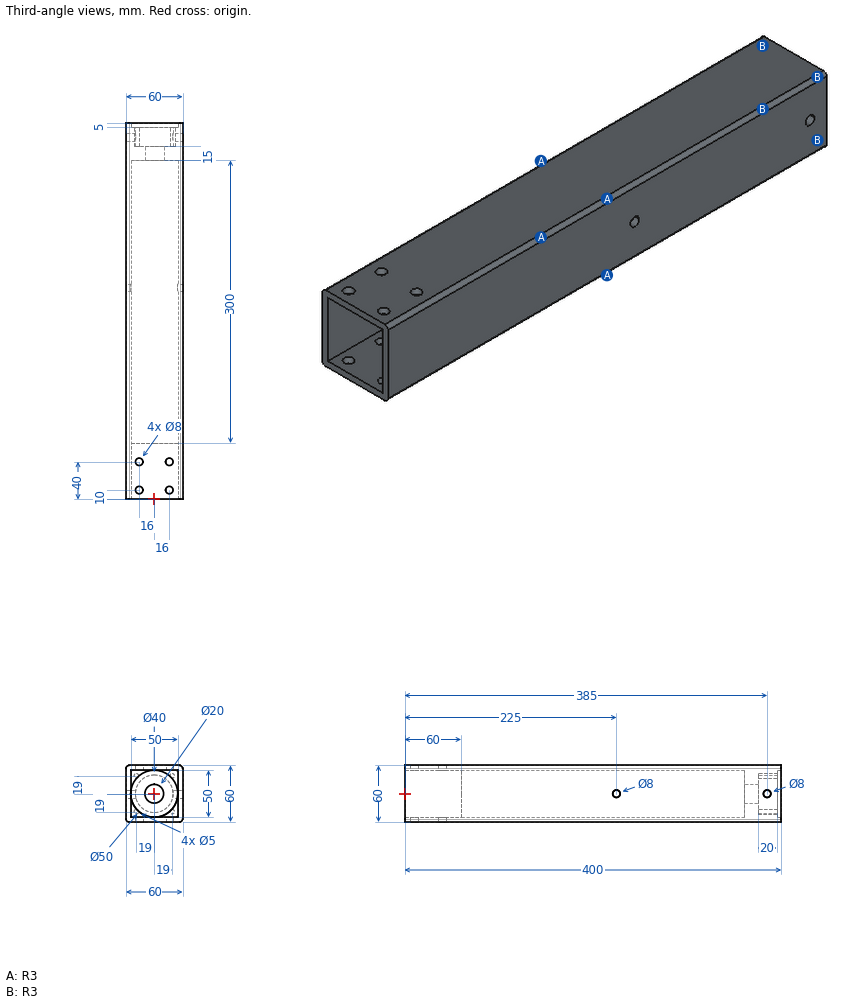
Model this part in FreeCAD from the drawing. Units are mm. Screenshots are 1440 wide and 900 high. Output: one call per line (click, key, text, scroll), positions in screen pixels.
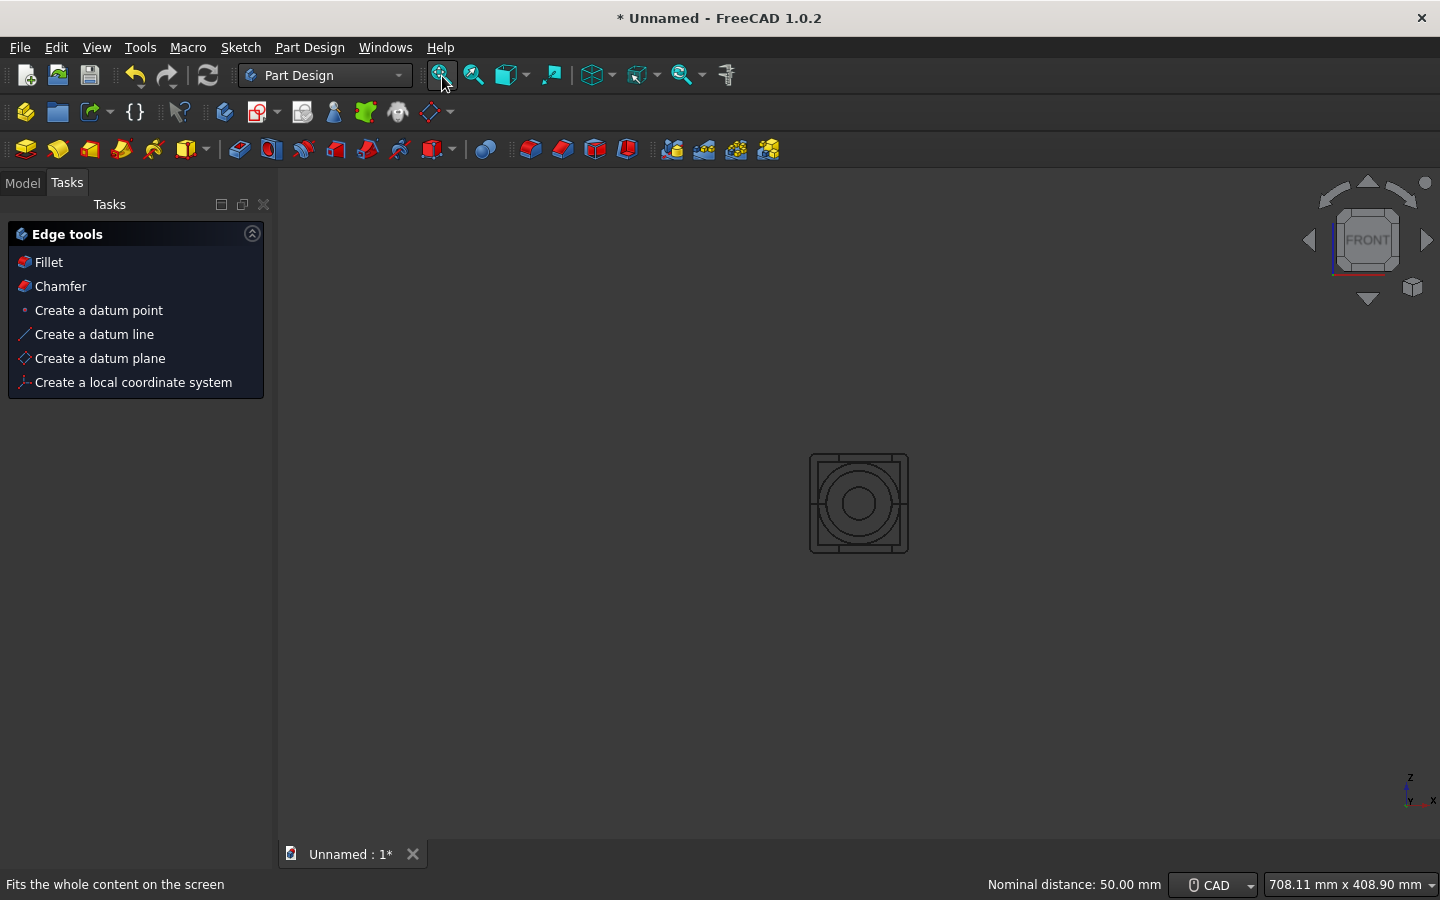
click(442, 76)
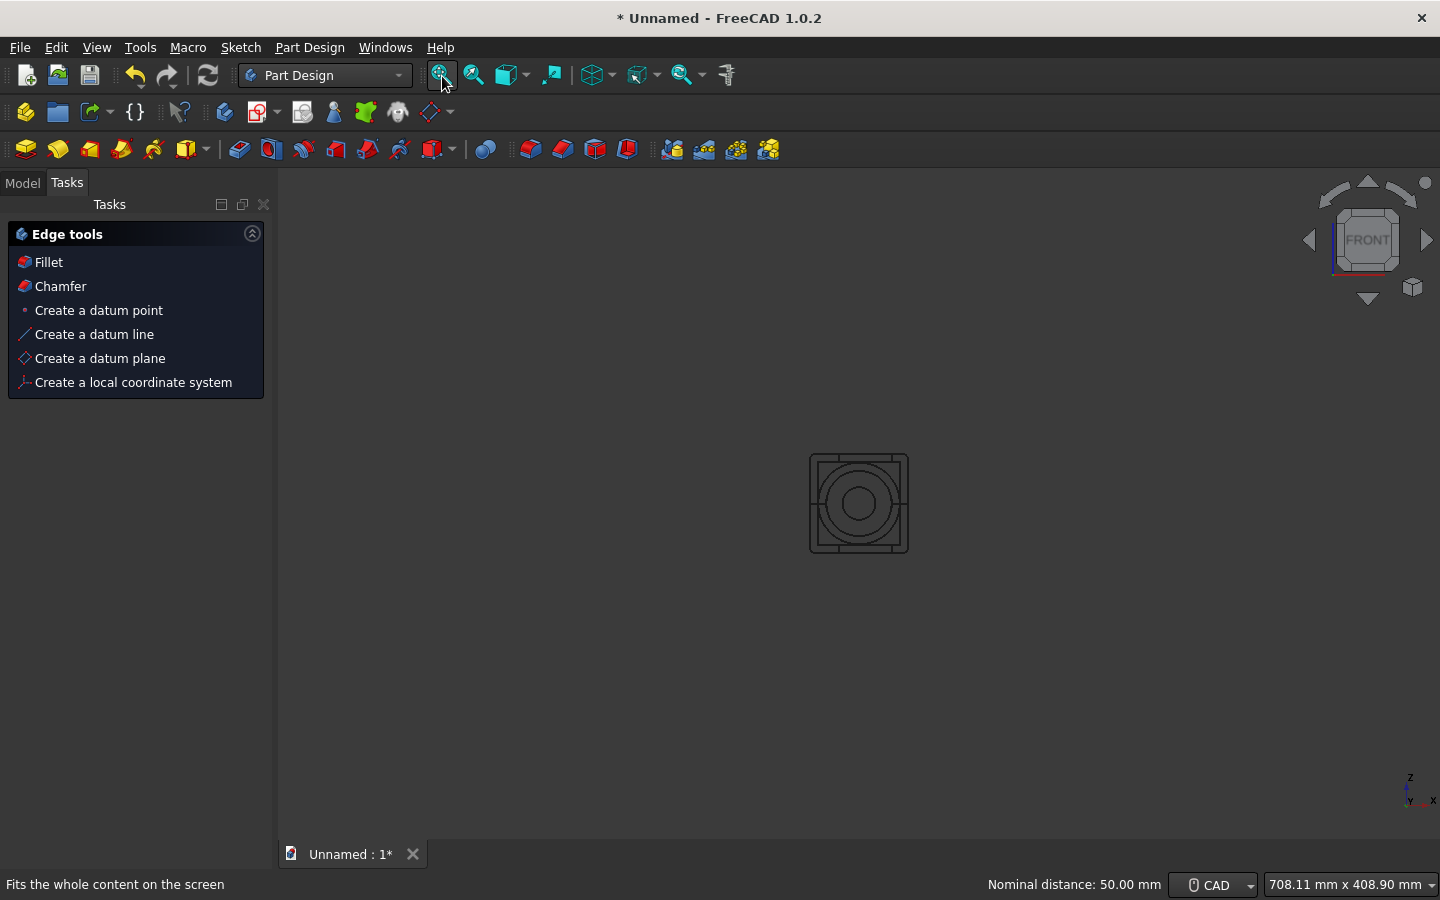
scroll(900, 461, up, 8)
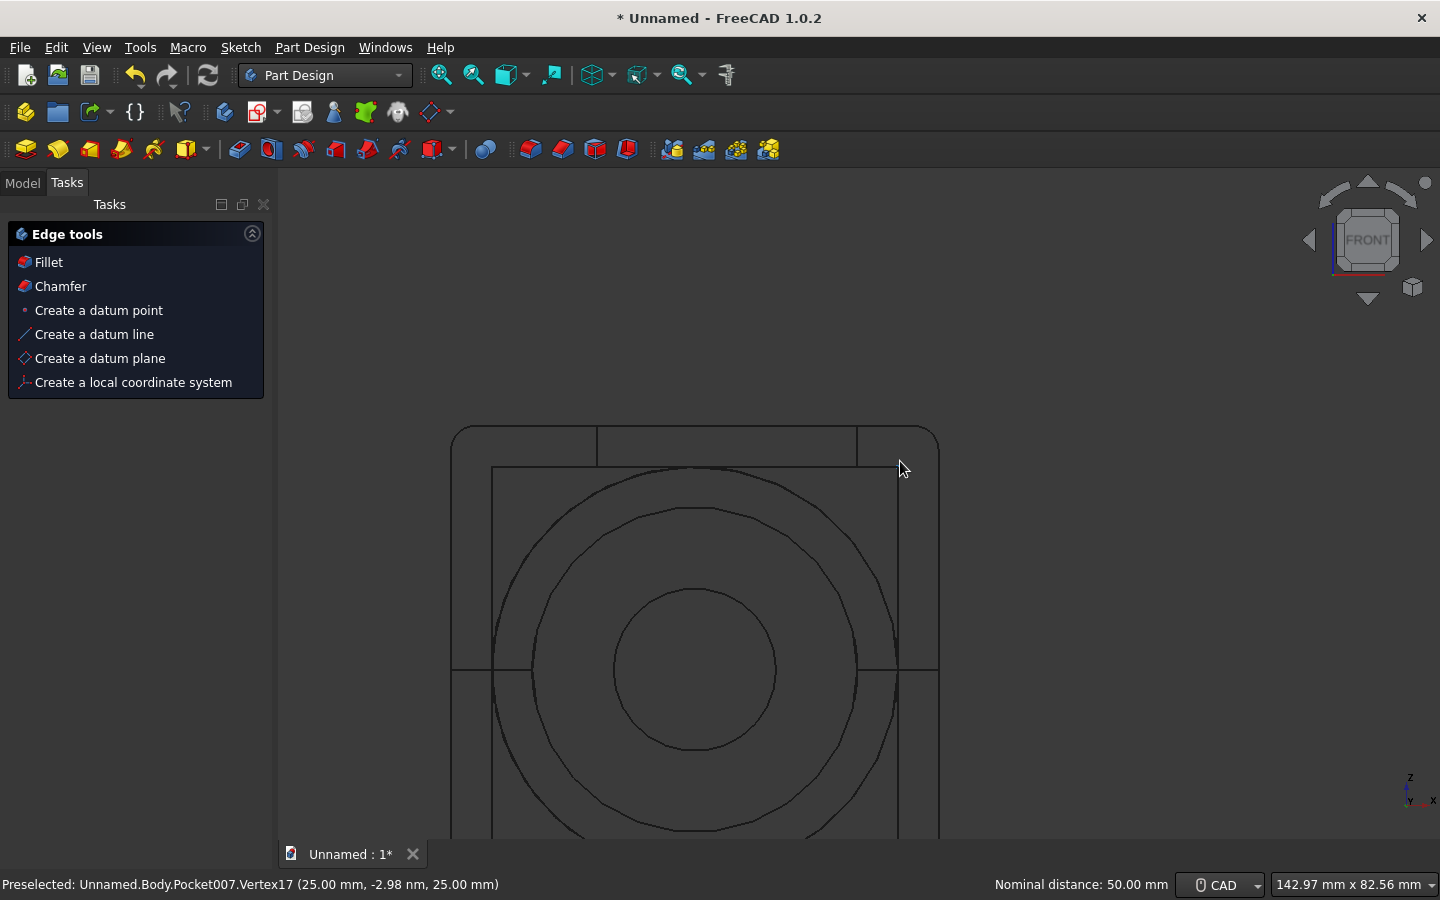
click(442, 76)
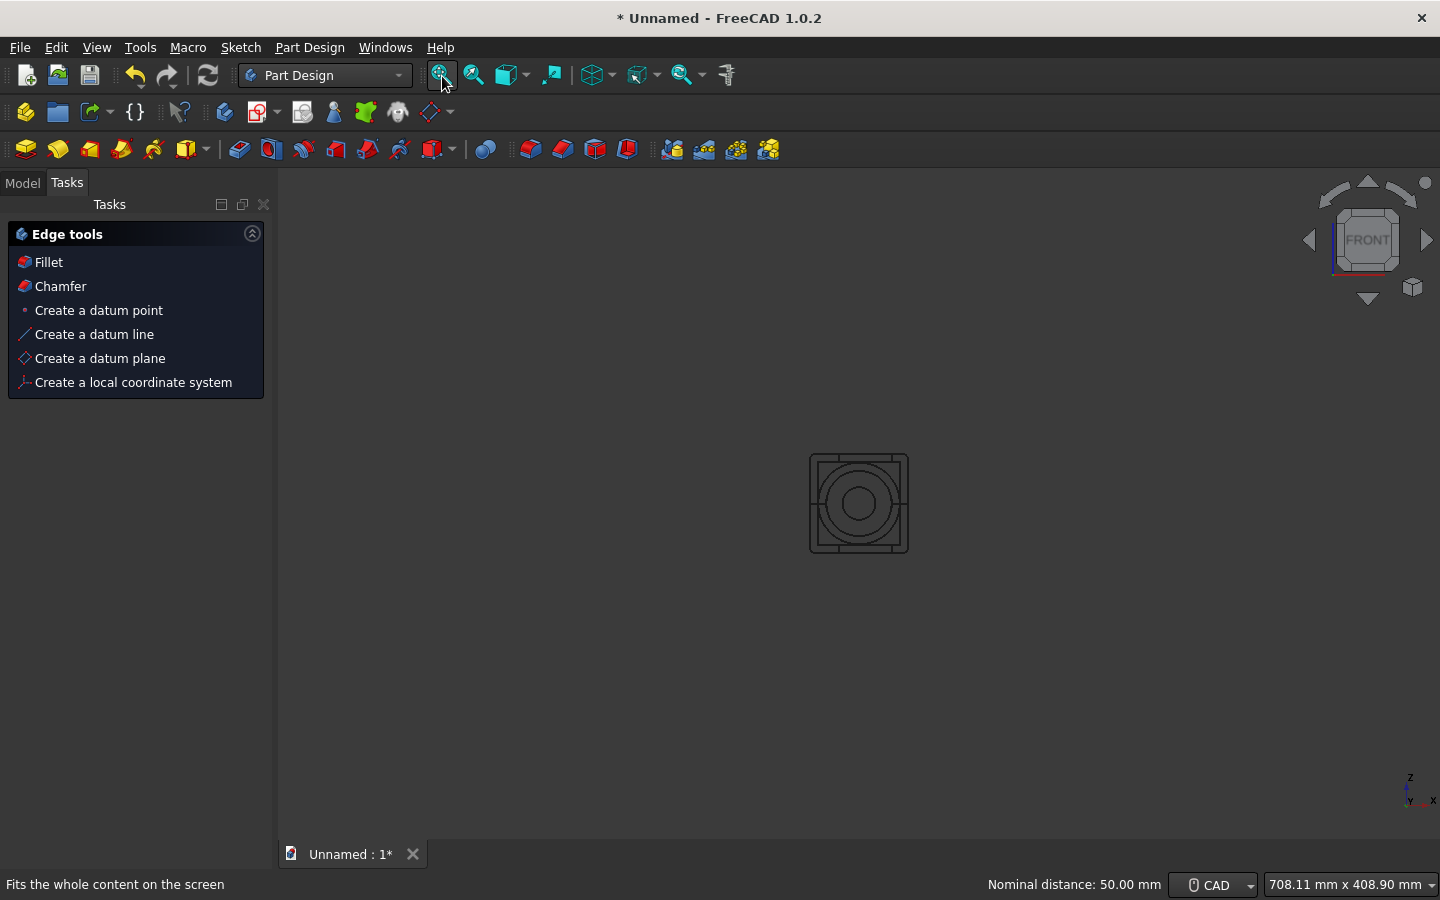
key(3)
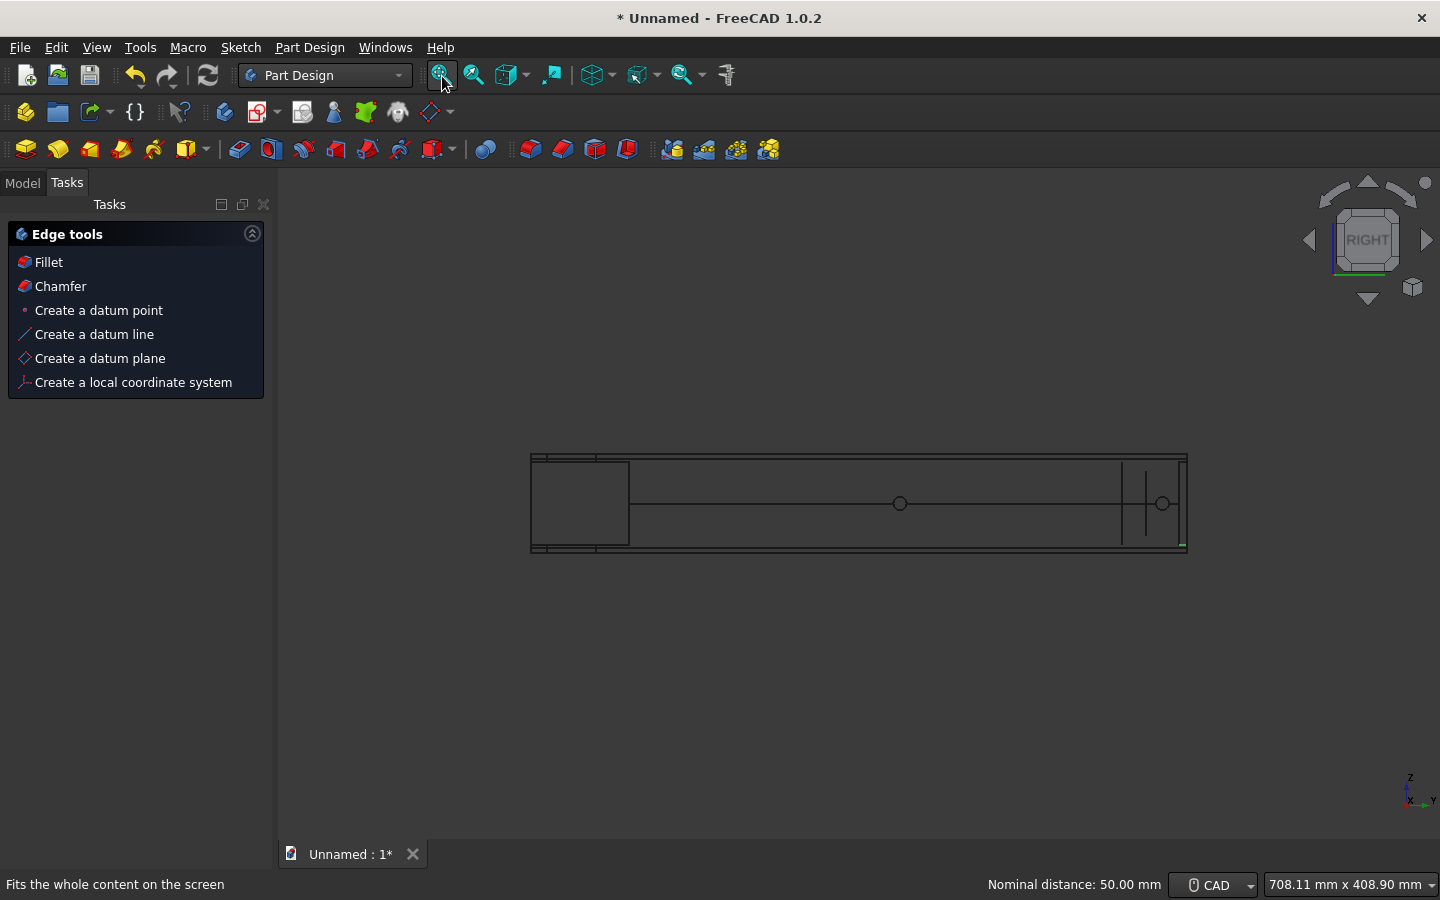
scroll(1183, 461, up, 8)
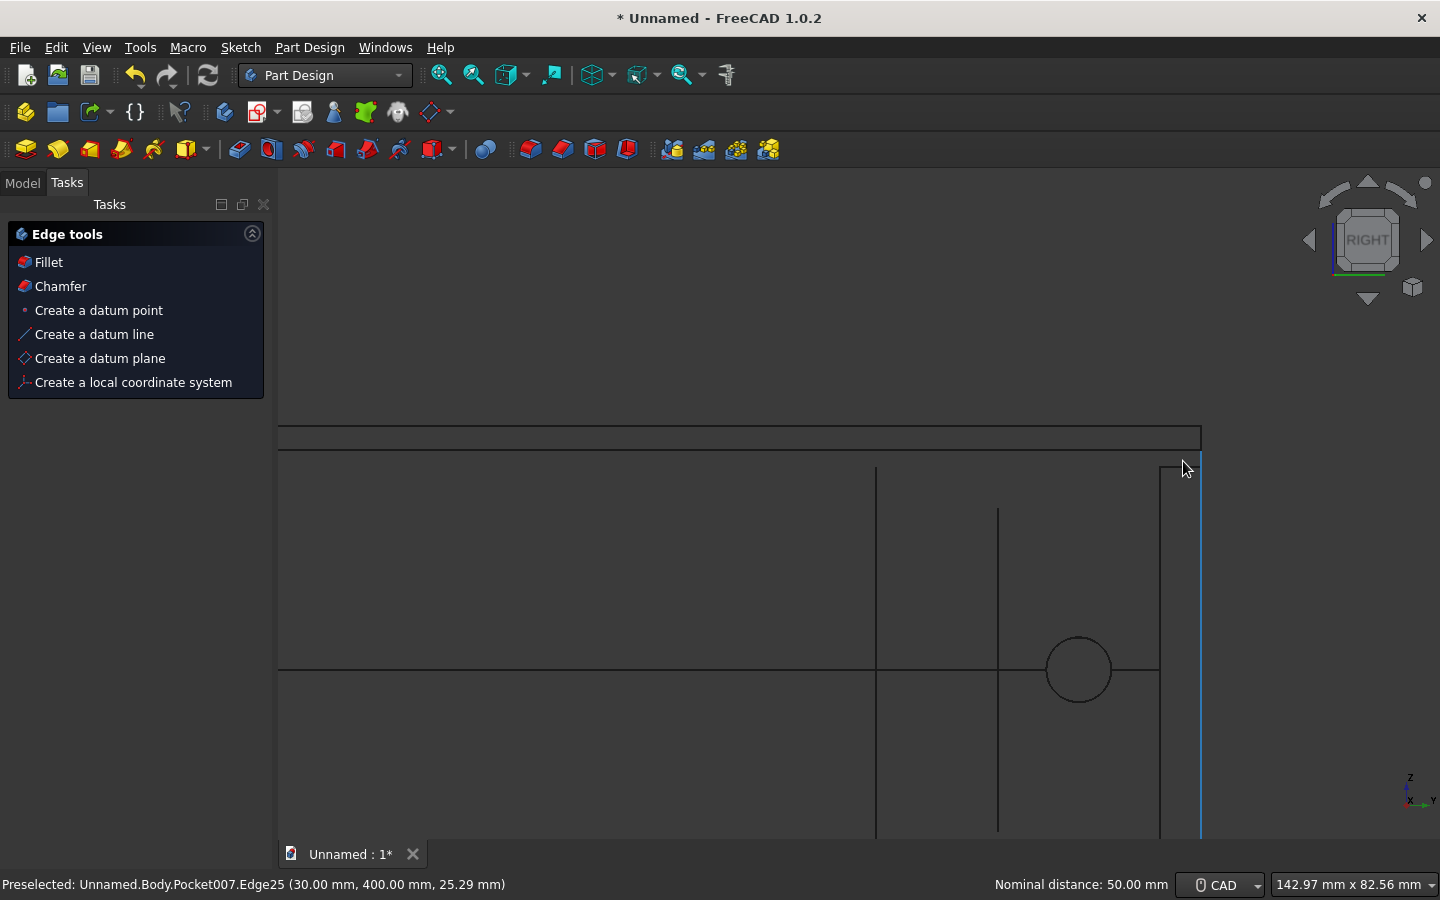
click(1180, 466, ctrl)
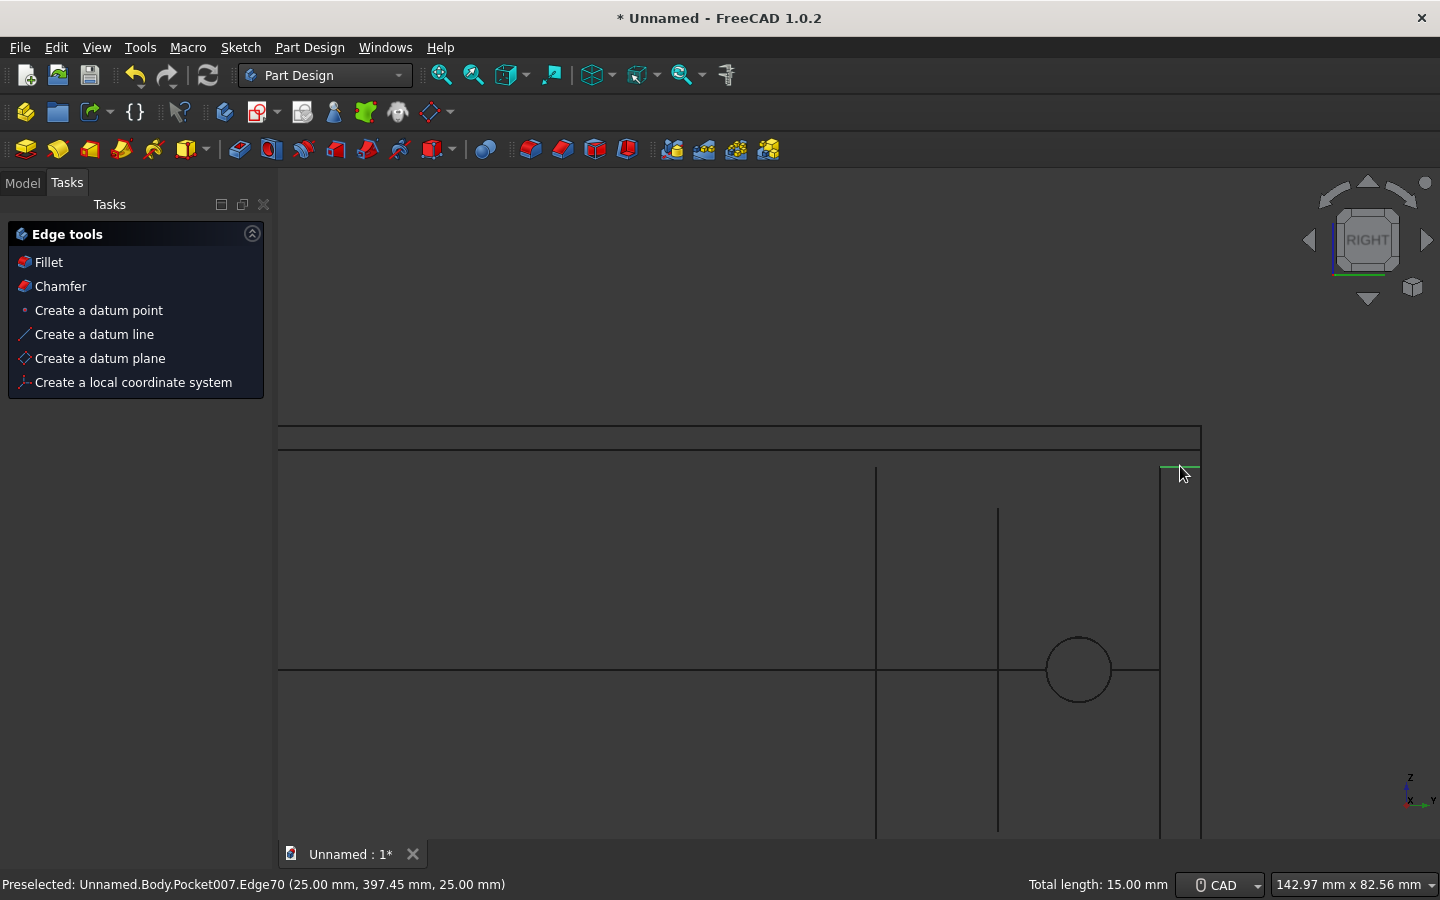
key(v)
key(f)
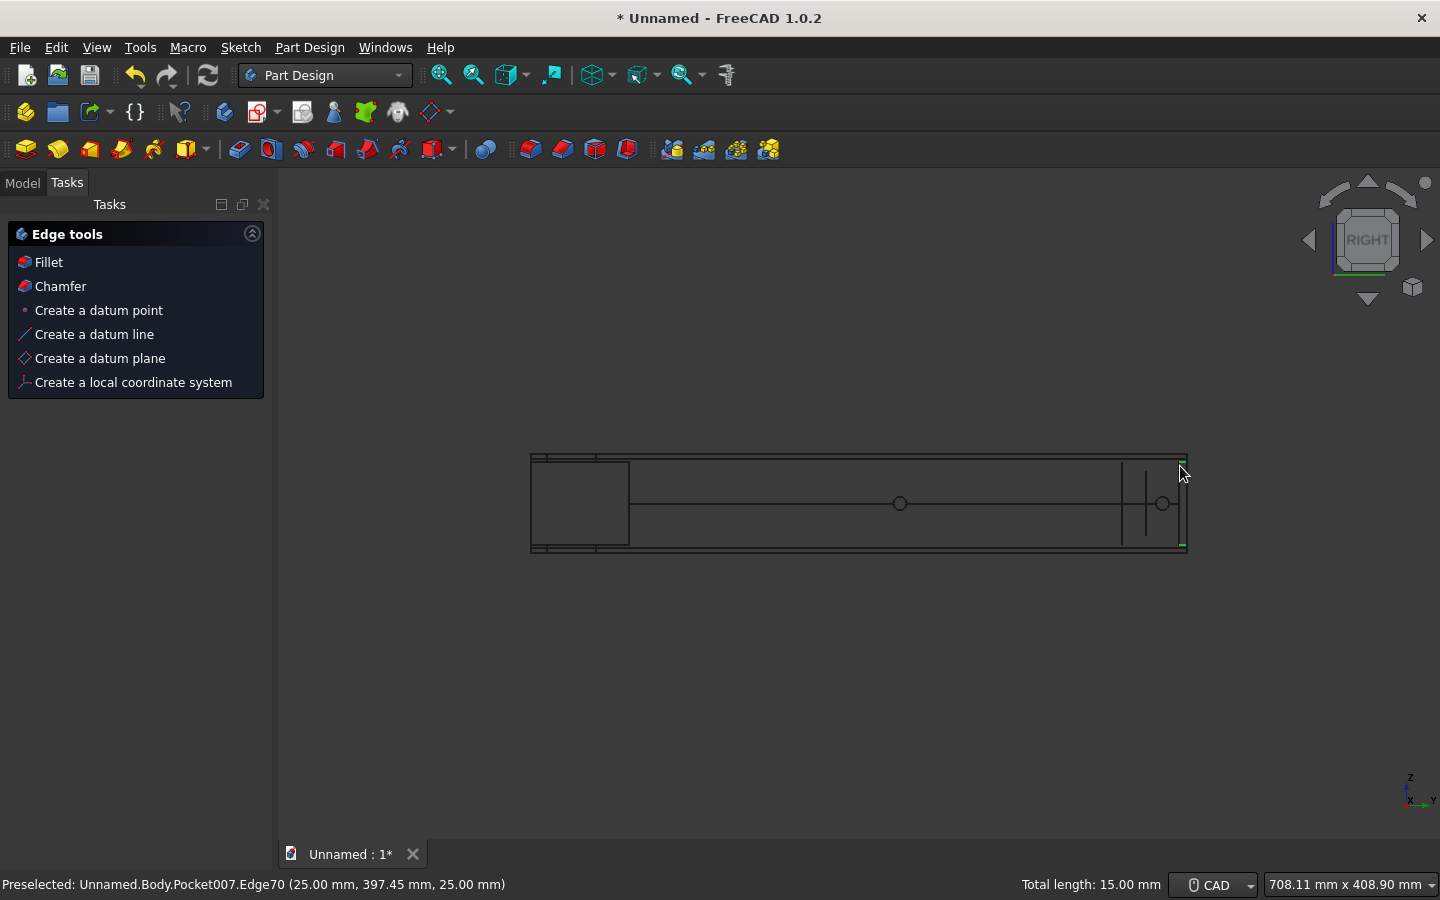
key(5)